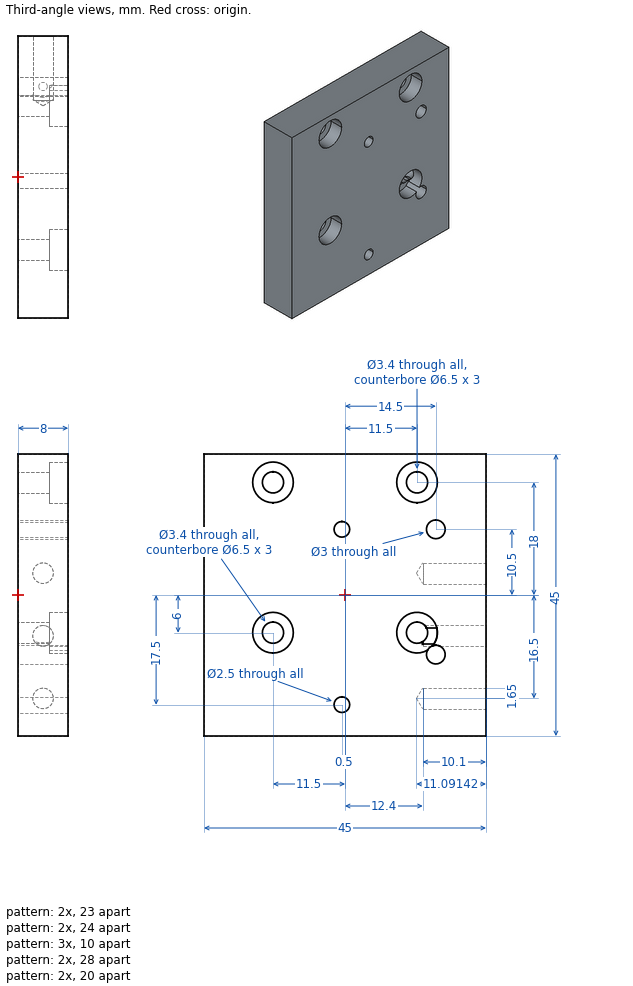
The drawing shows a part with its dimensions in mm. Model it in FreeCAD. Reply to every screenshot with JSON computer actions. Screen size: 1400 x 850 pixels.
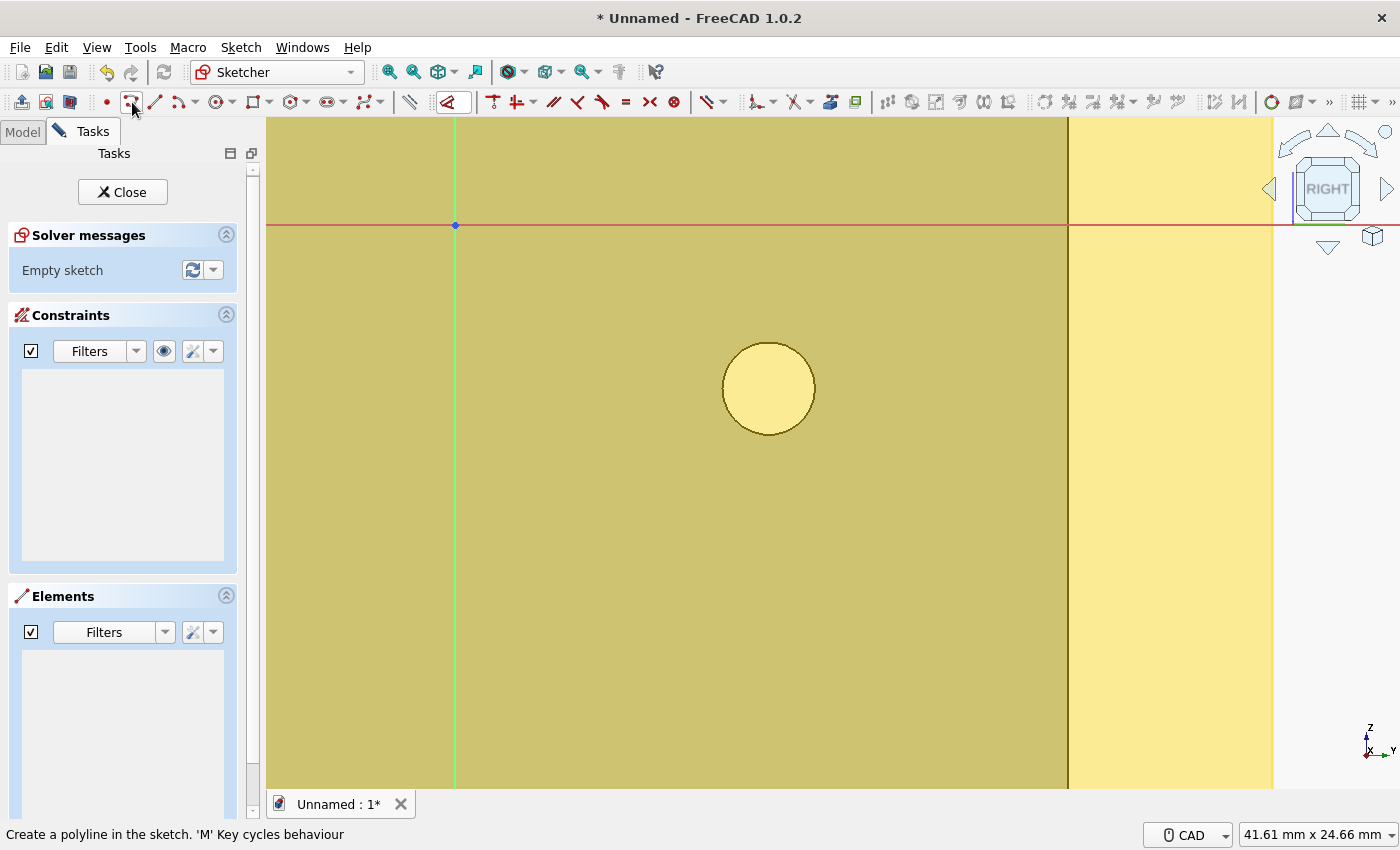
{"action": "left_click", "coordinate": [793, 630]}
{"action": "left_click", "coordinate": [766, 675]}
{"action": "left_click", "coordinate": [1068, 675]}
{"action": "left_click", "coordinate": [1068, 630]}
{"action": "left_click", "coordinate": [793, 631]}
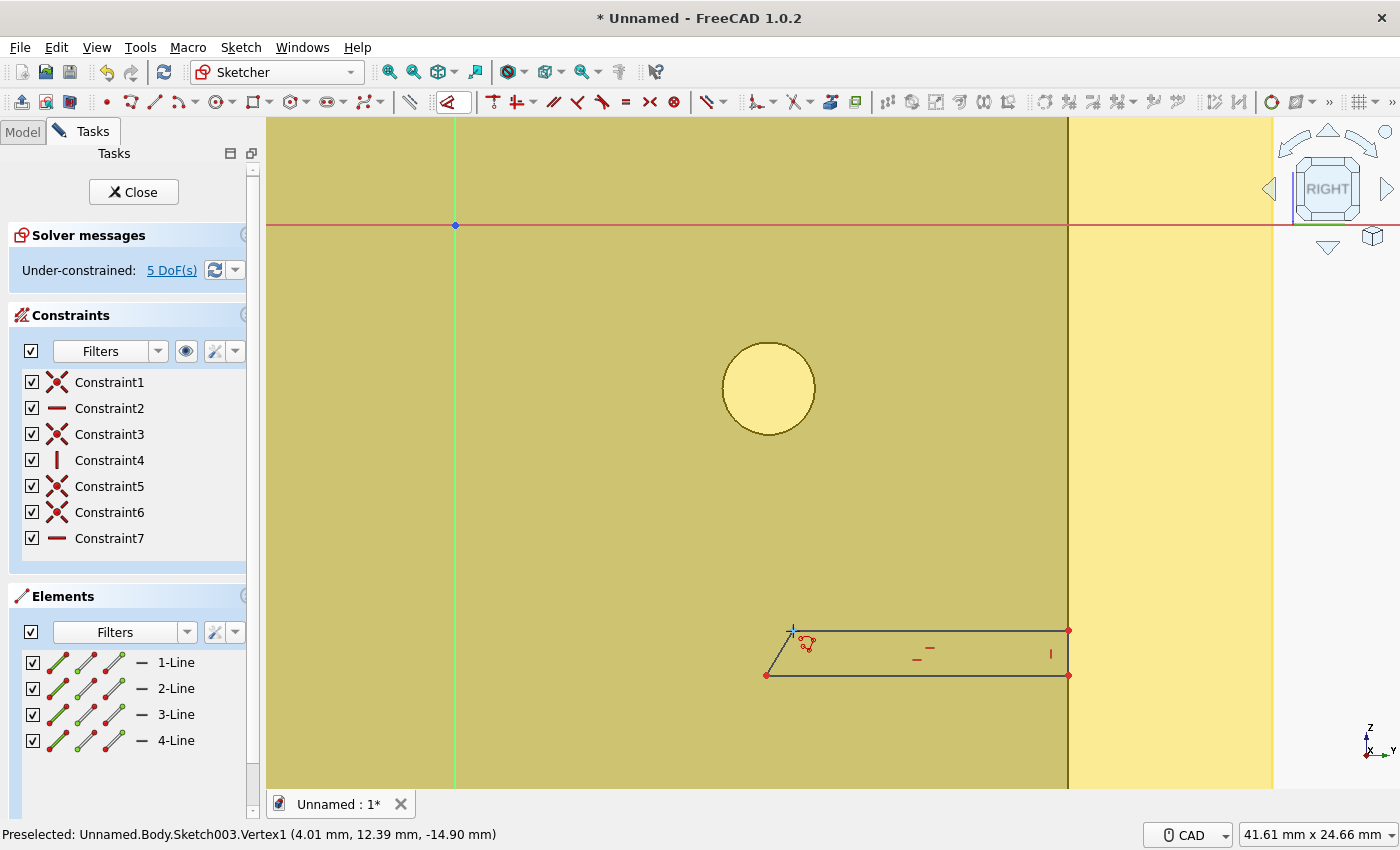
{"action": "key", "text": "g l"}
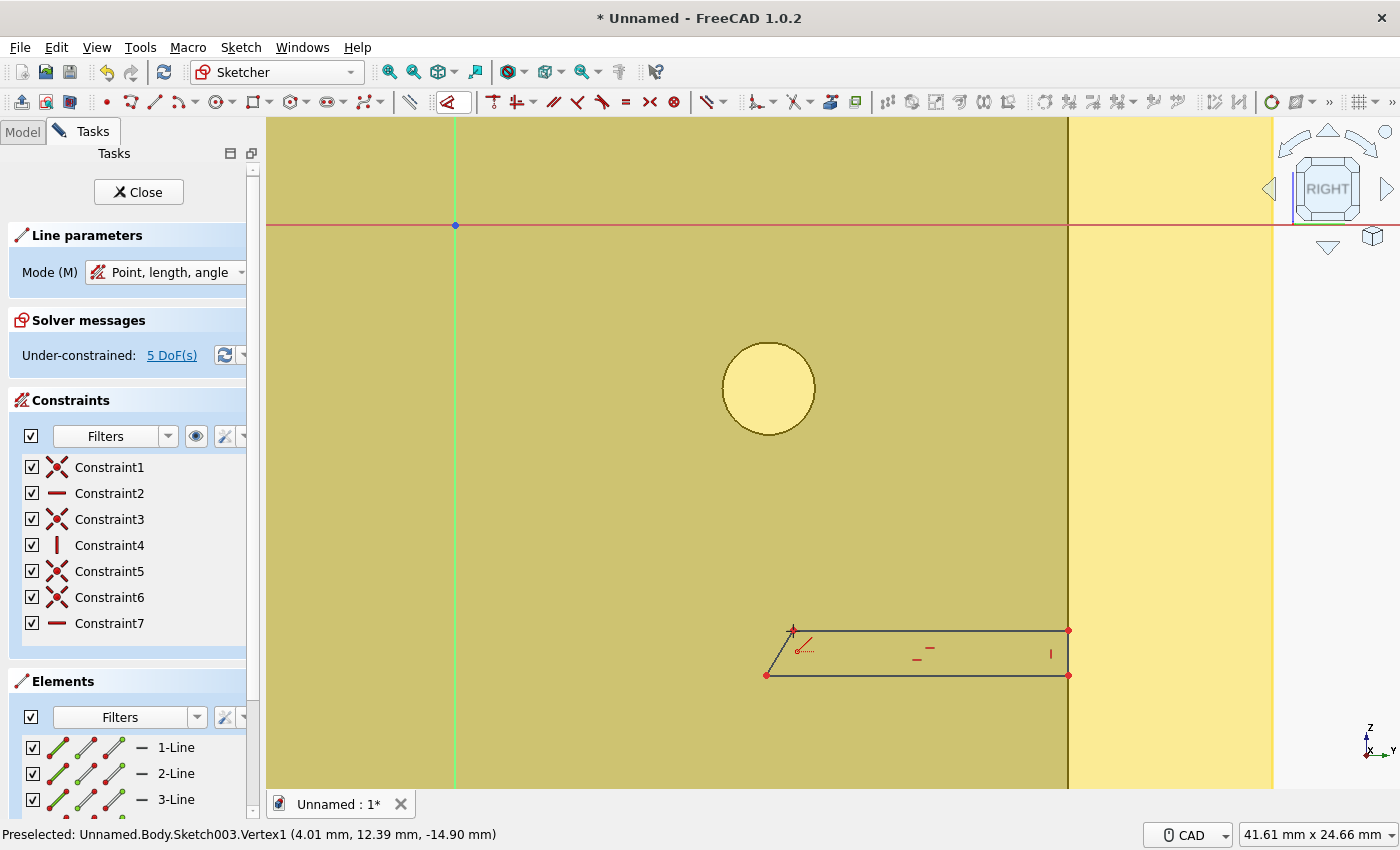
{"action": "left_click", "coordinate": [736, 675]}
{"action": "left_click", "coordinate": [645, 675]}
{"action": "key", "text": "Escape"}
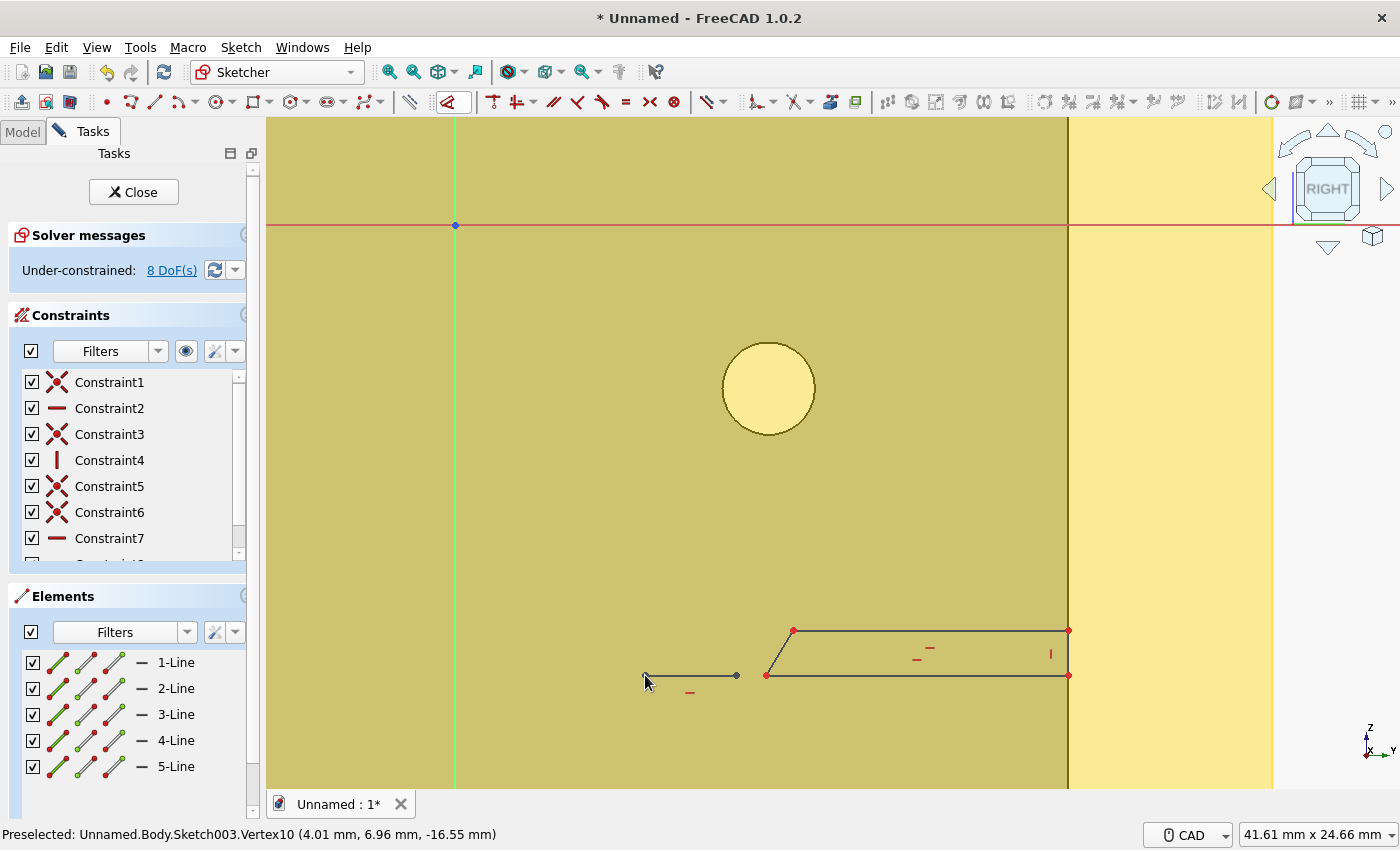
{"action": "left_click", "coordinate": [709, 676]}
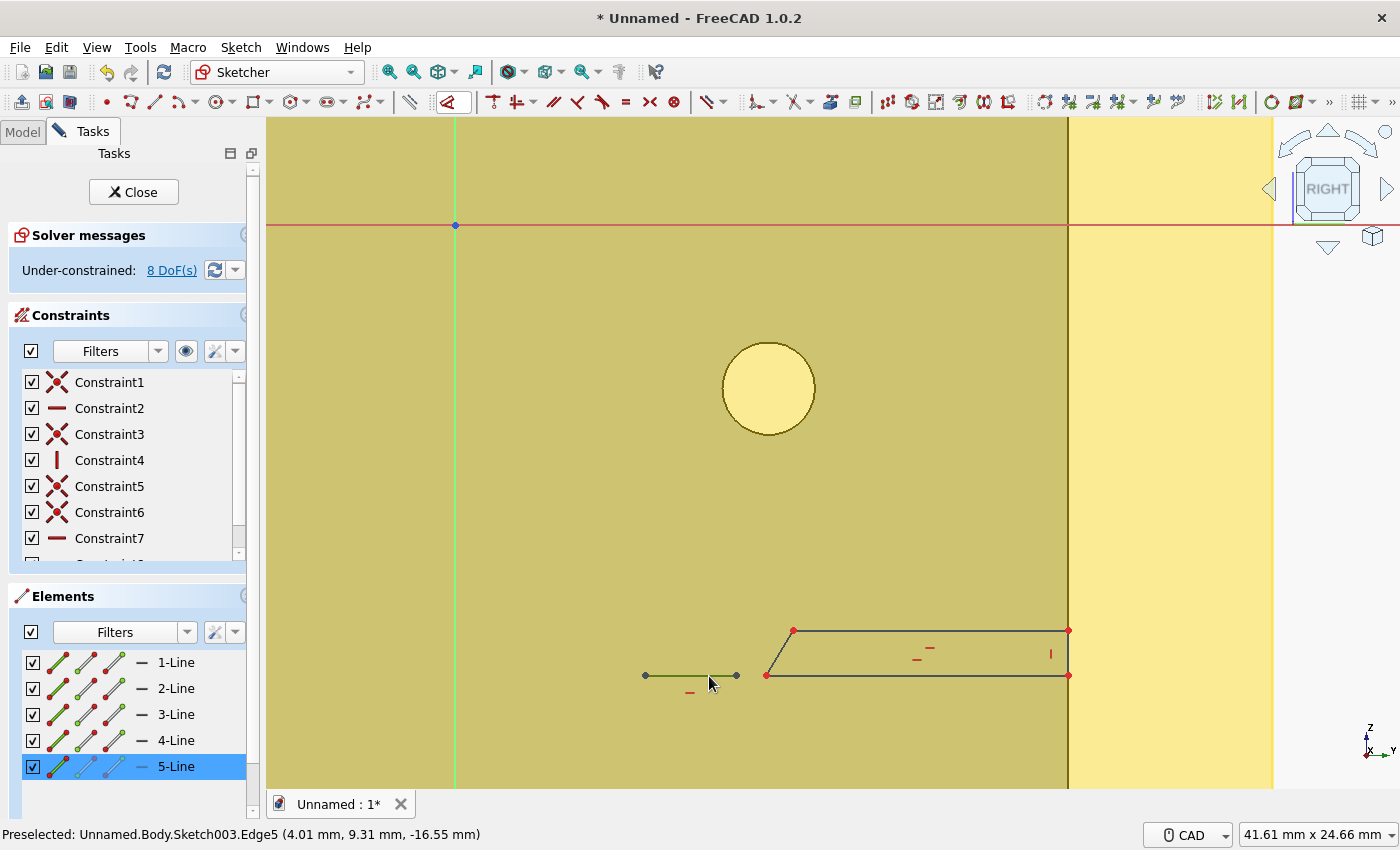
{"action": "key", "text": "g n"}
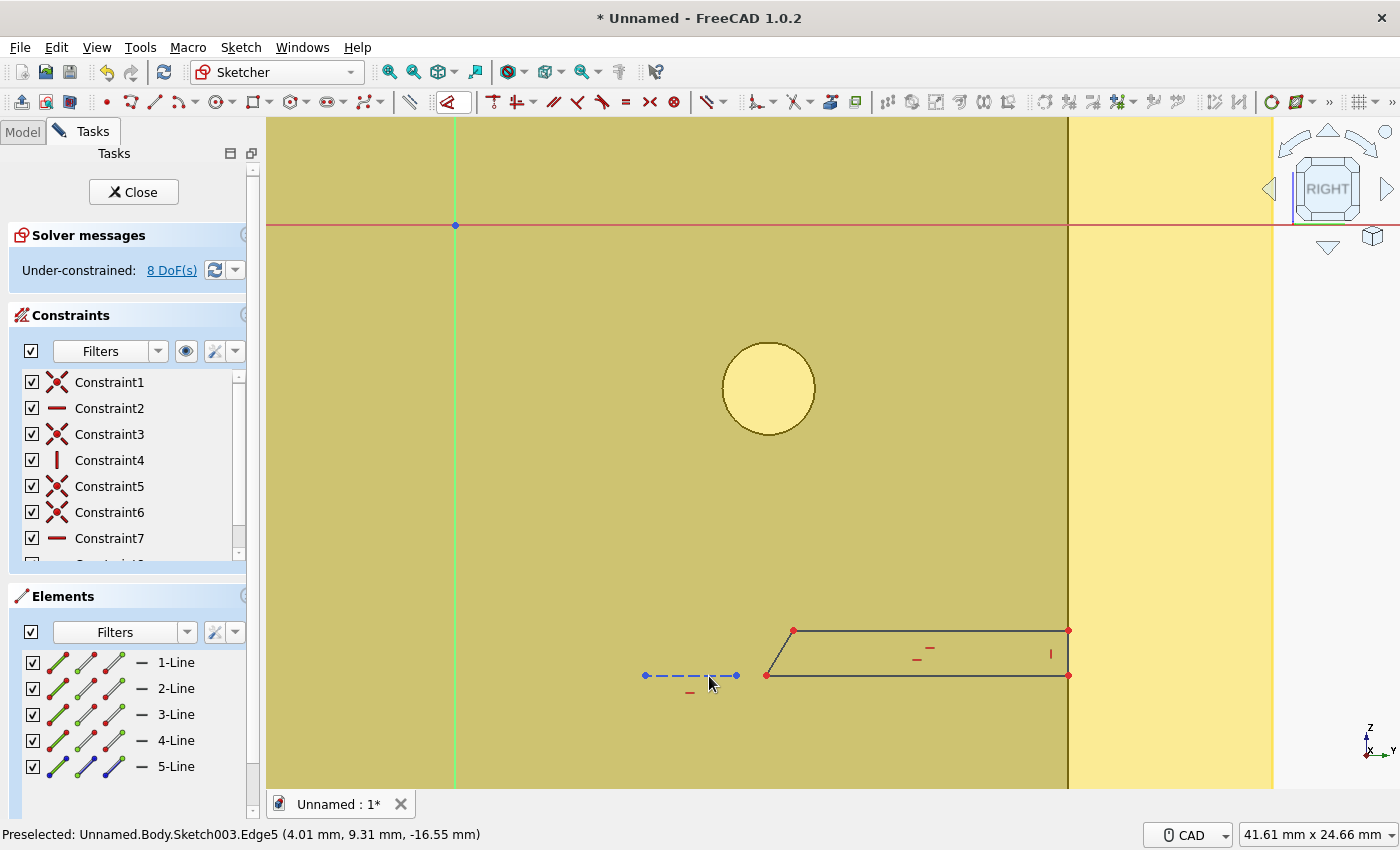
{"action": "key", "text": "d"}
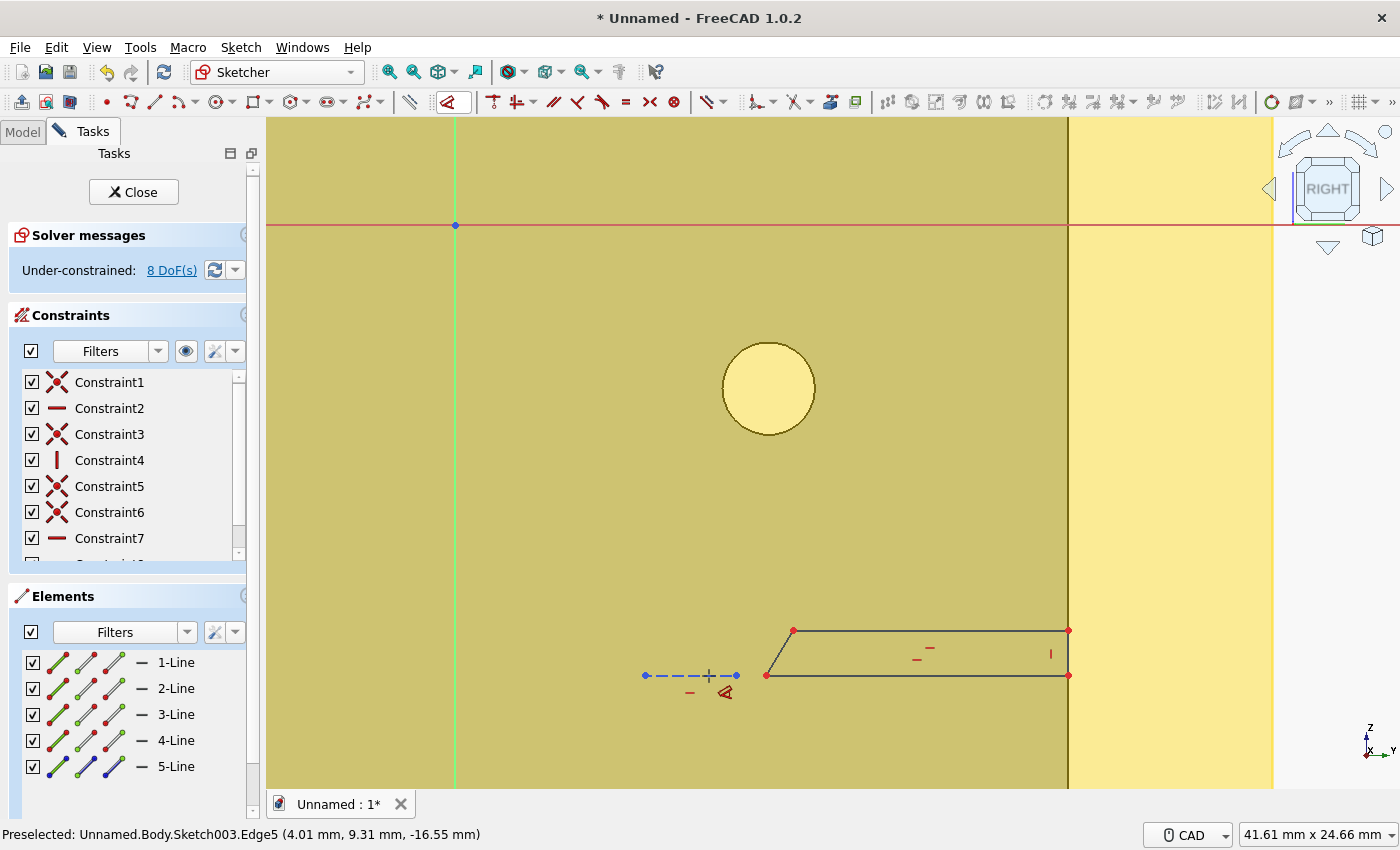
{"action": "left_click", "coordinate": [1068, 662]}
{"action": "left_click", "coordinate": [1102, 654]}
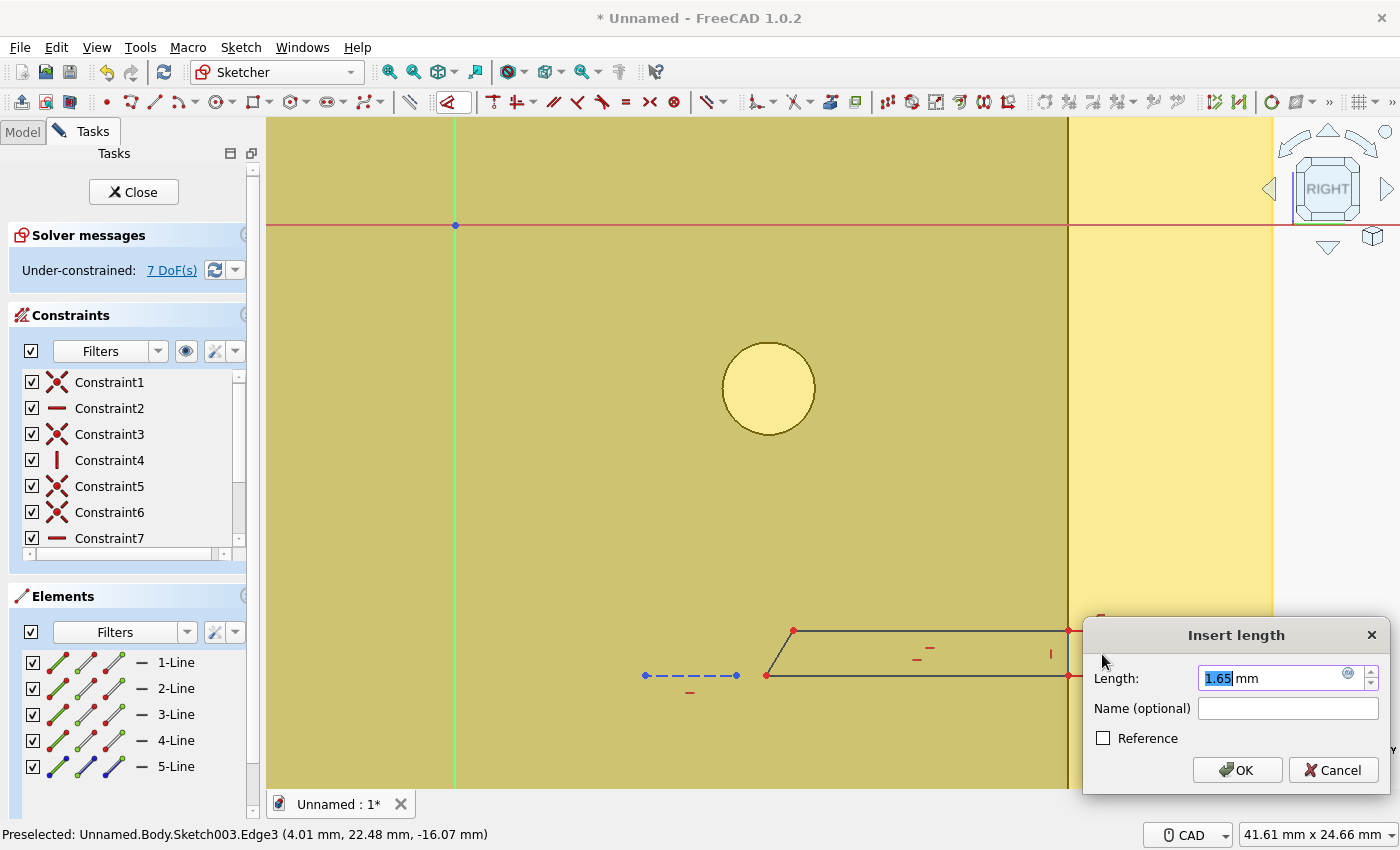
{"action": "type", "text": "1.65"}
{"action": "key", "text": "Return"}